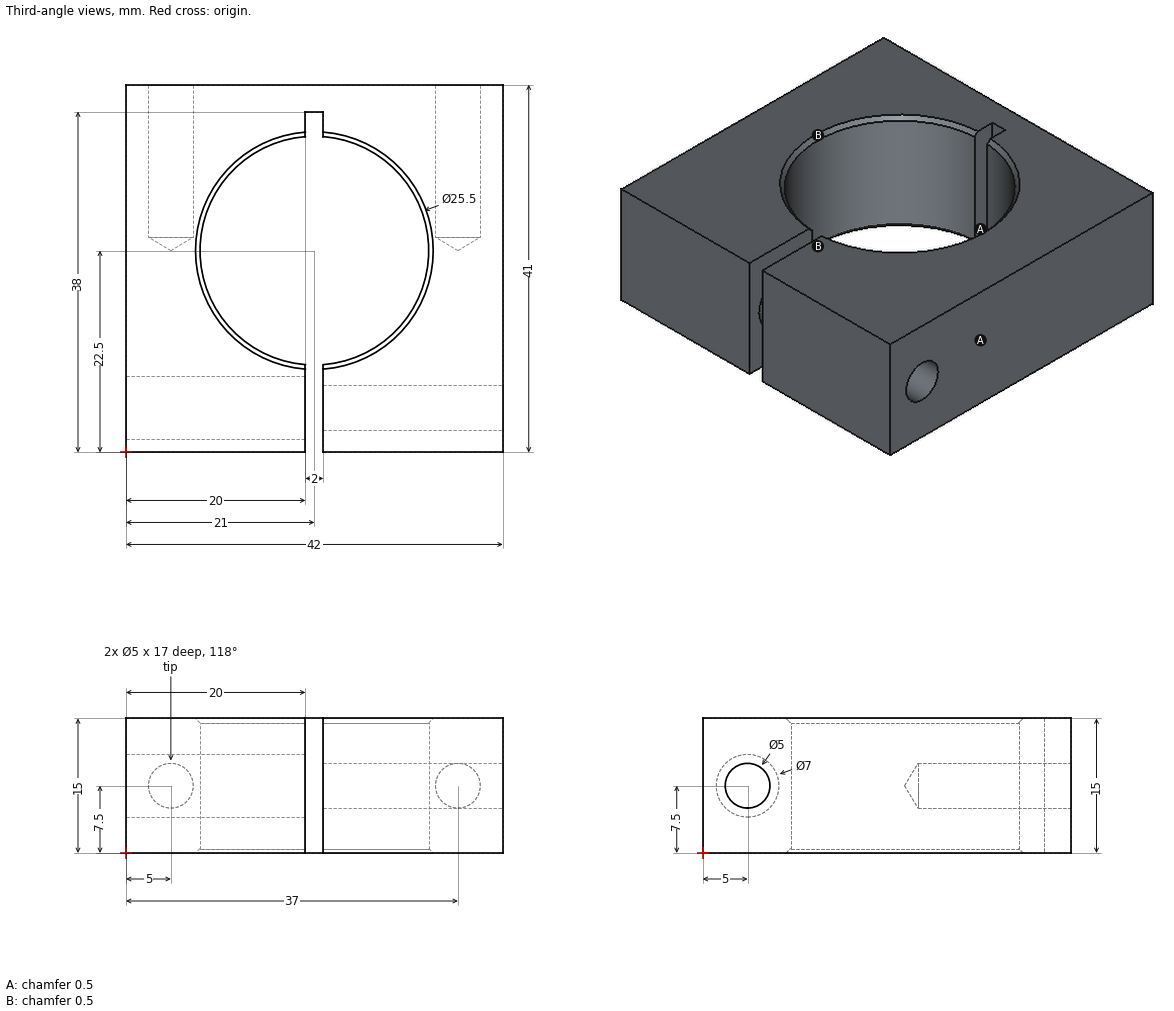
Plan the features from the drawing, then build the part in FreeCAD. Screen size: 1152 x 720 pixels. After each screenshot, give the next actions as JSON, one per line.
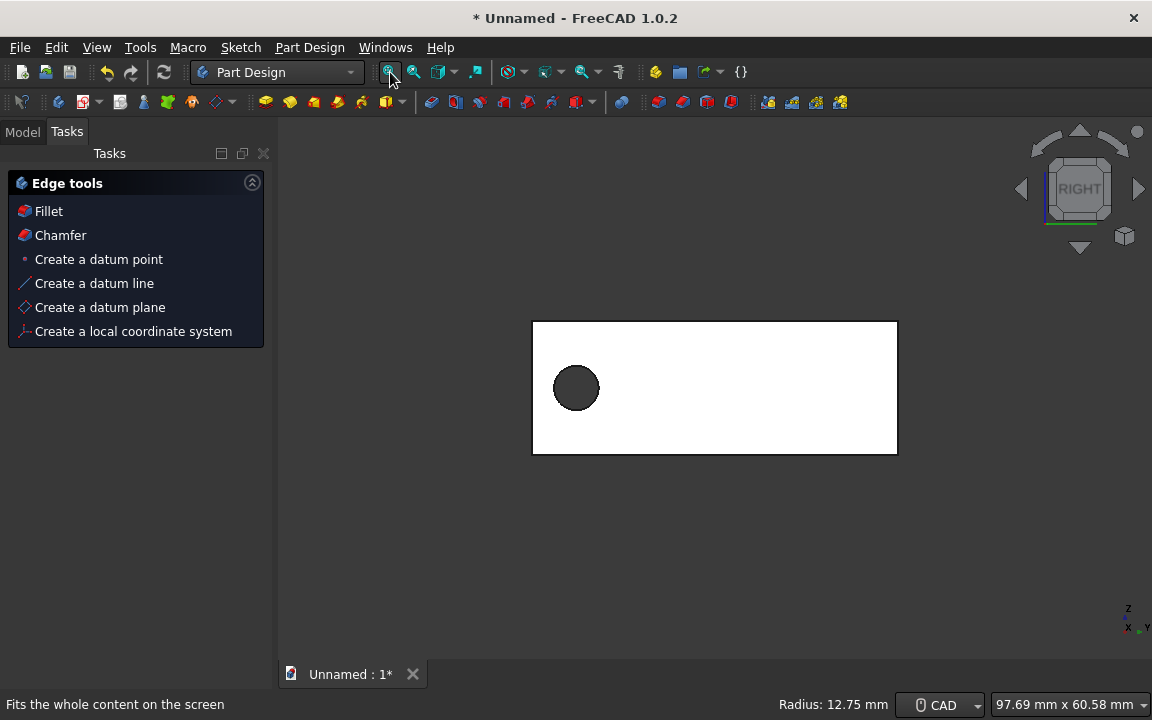
{"action": "left_click", "coordinate": [390, 72]}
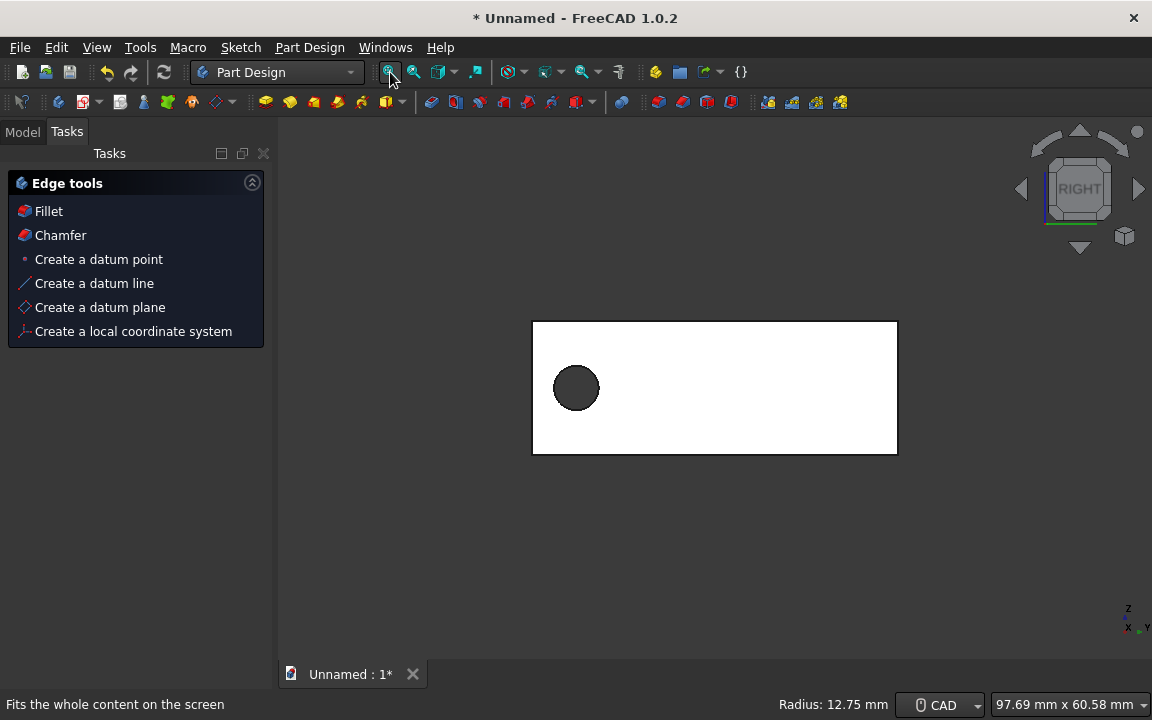
{"action": "key", "text": "5"}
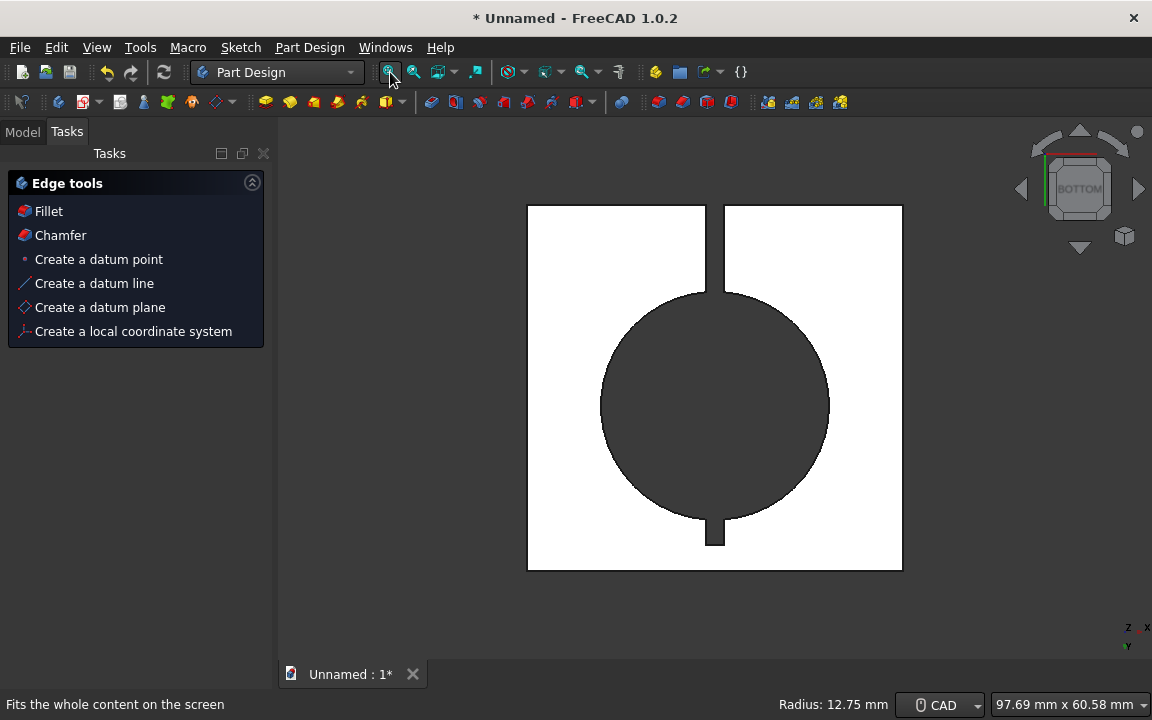
{"action": "left_click", "coordinate": [786, 316], "text": "ctrl"}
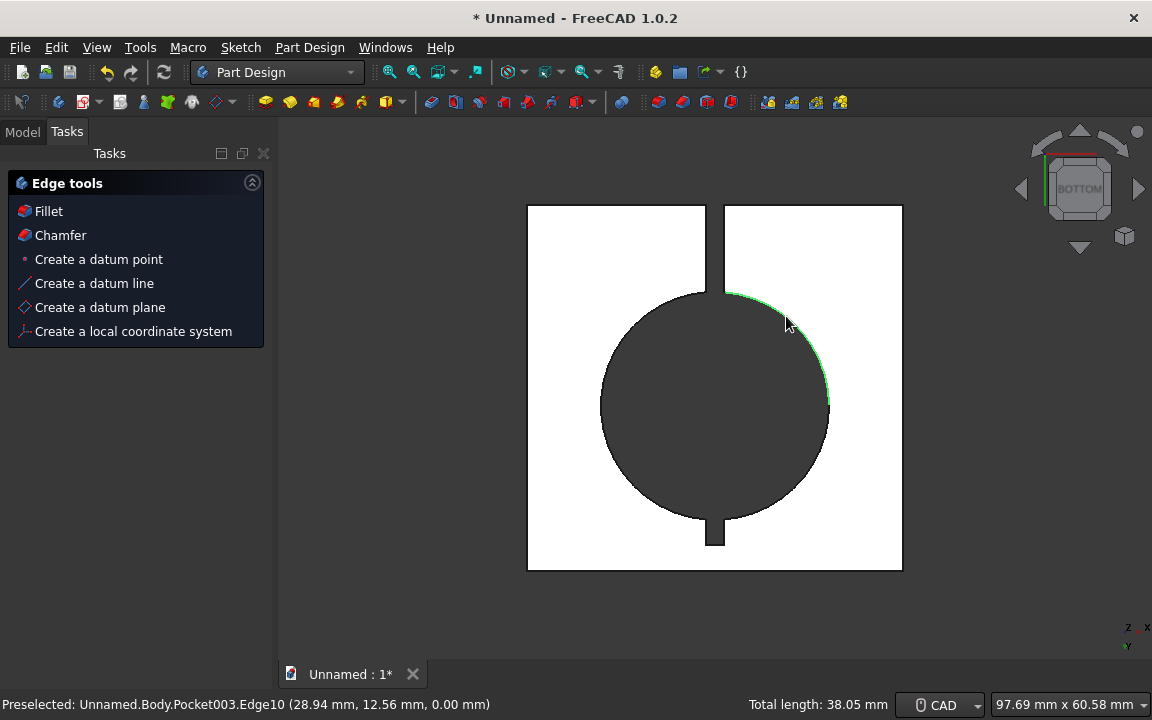
{"action": "left_click", "coordinate": [684, 102]}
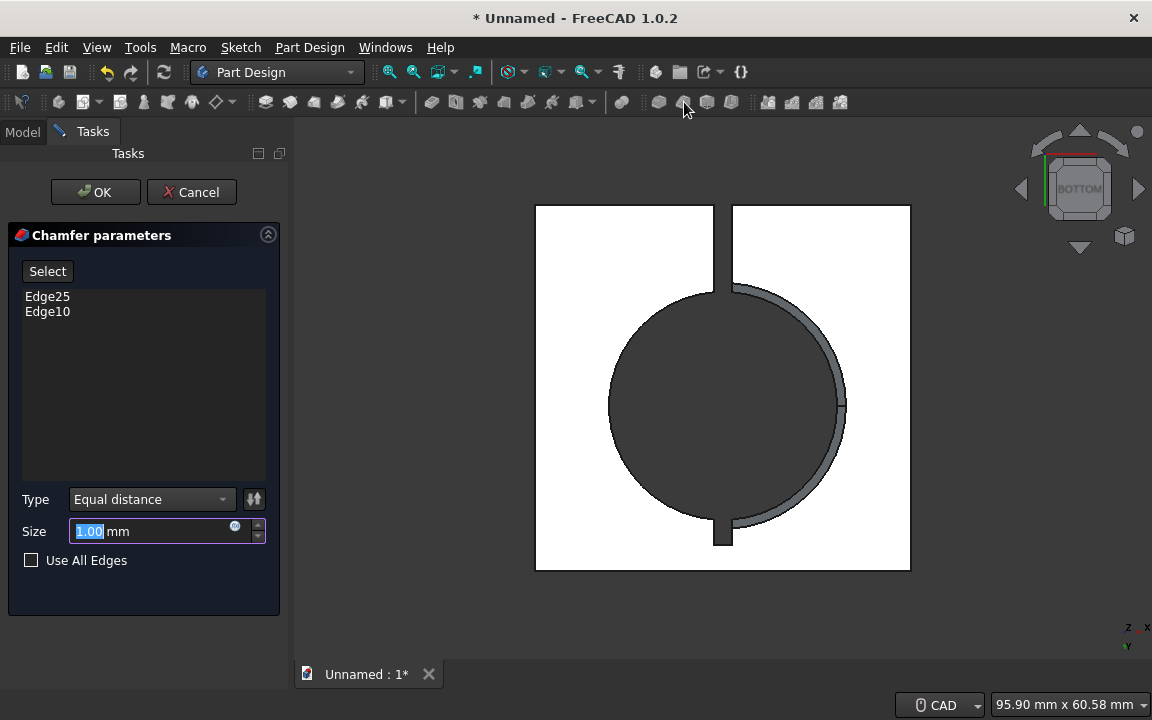
{"action": "type", "text": "0.5"}
{"action": "key", "text": "Tab"}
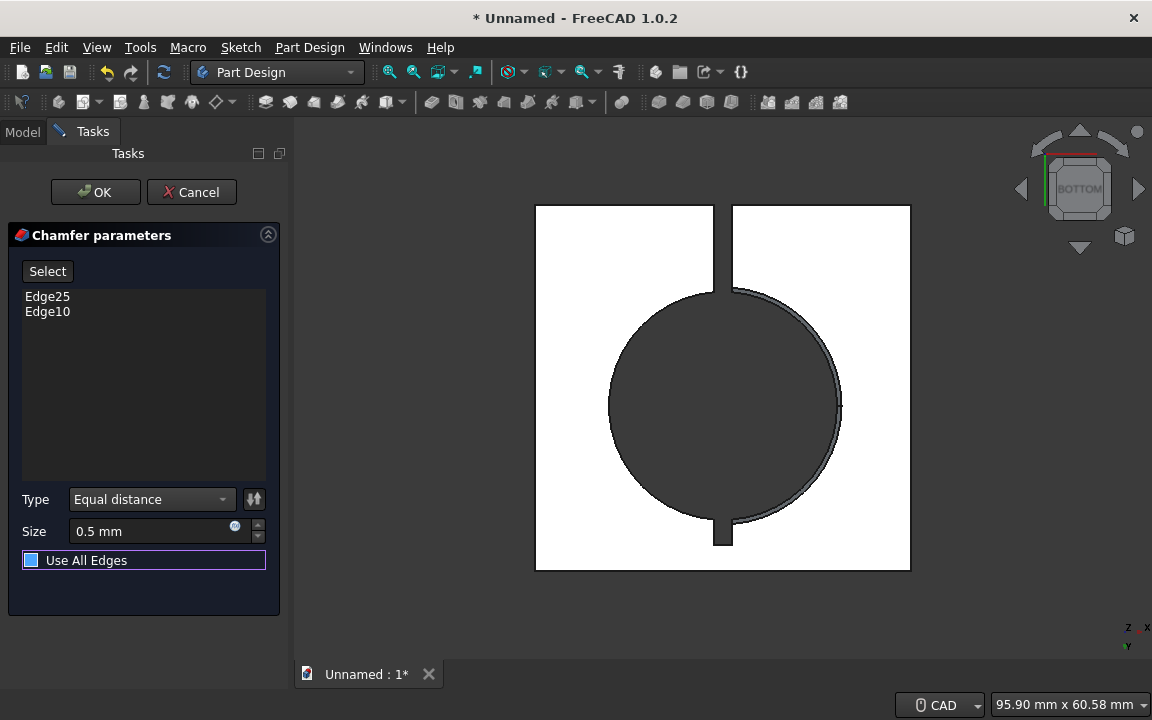
{"action": "left_click", "coordinate": [96, 192]}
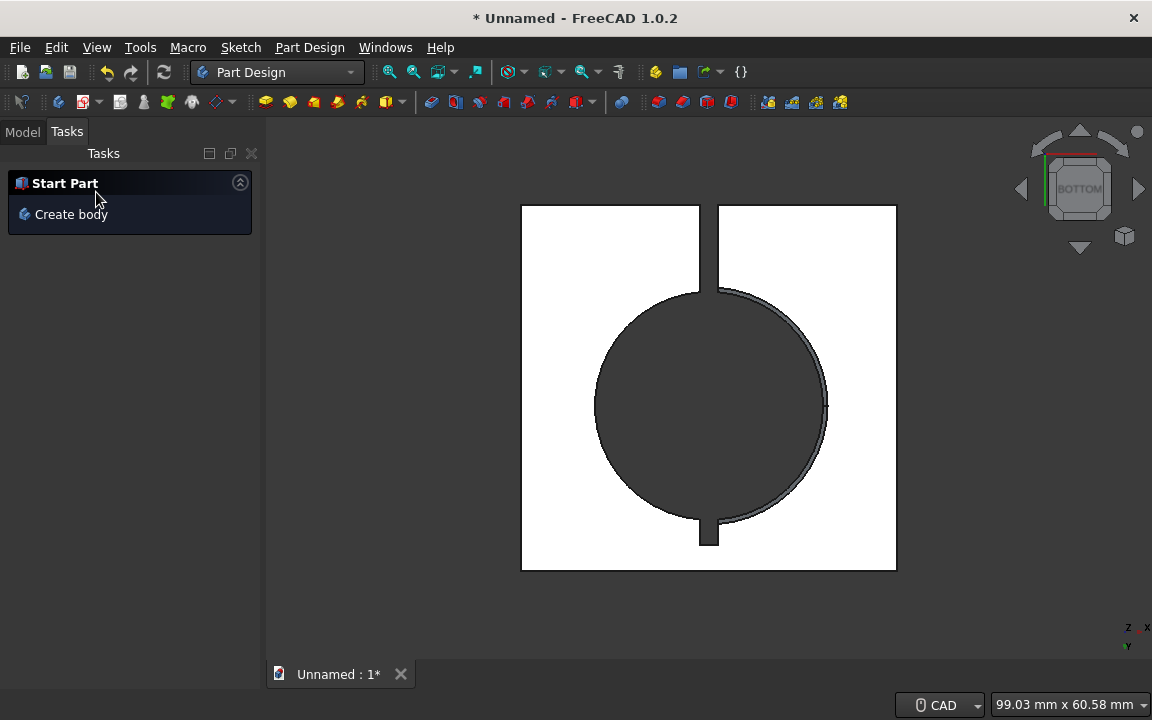
{"action": "left_click", "coordinate": [595, 405]}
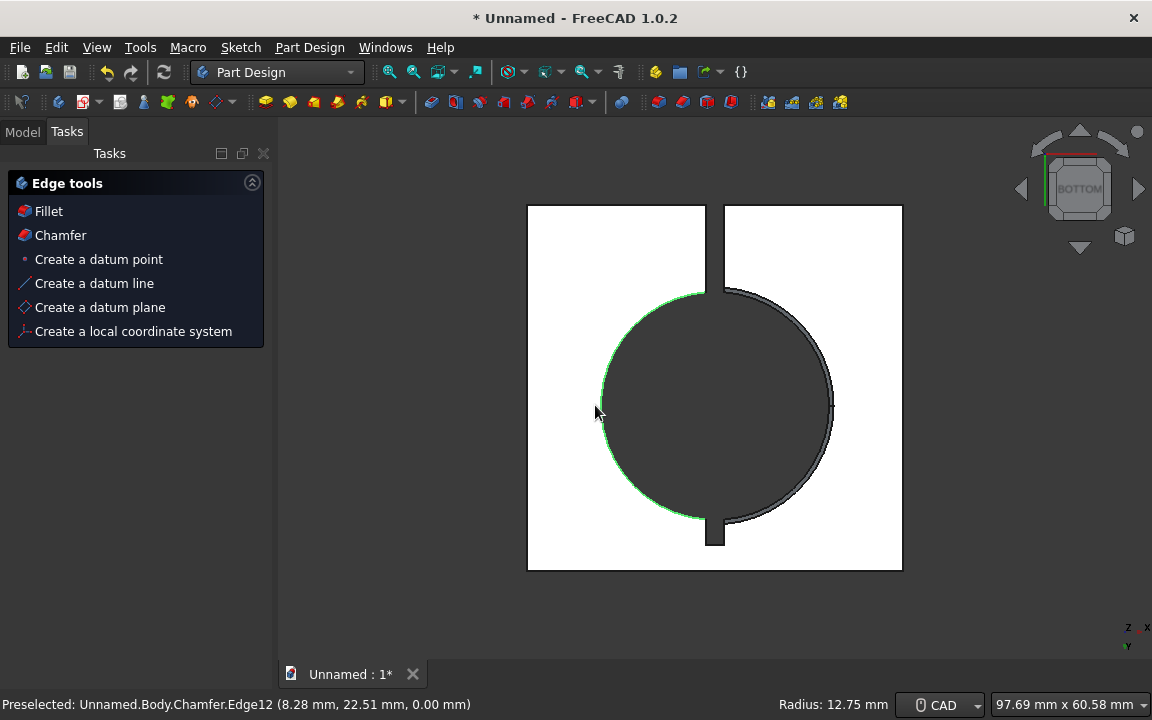
{"action": "key", "text": "0"}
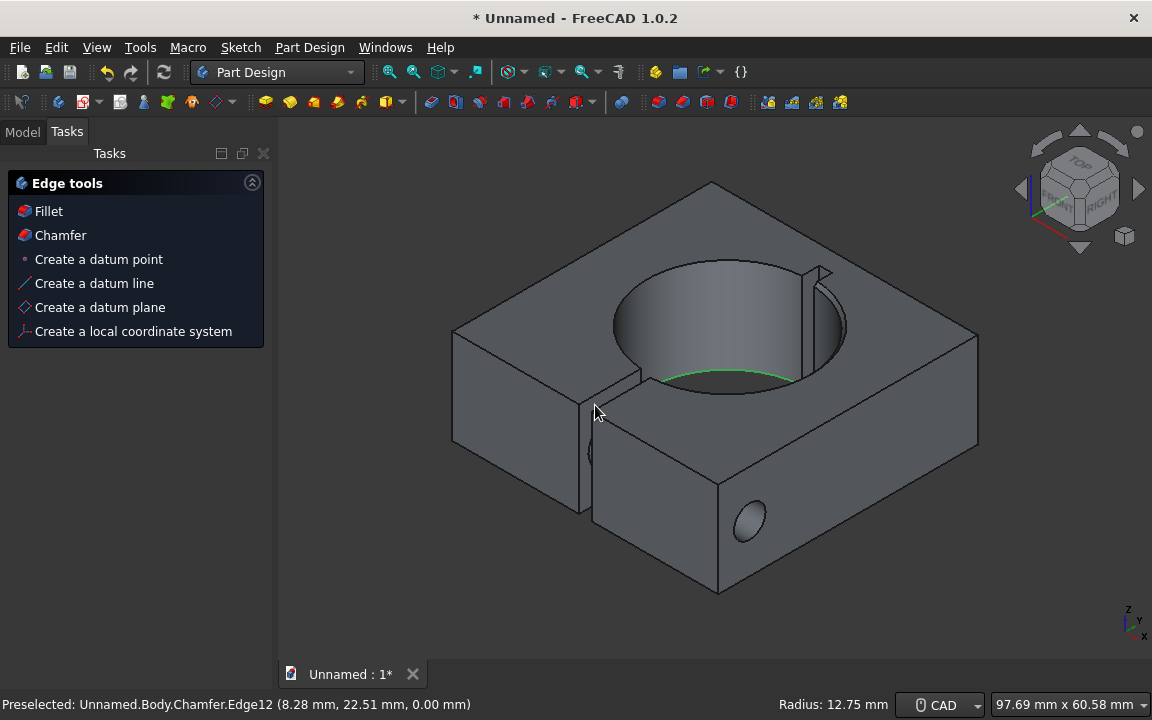
{"action": "left_click", "coordinate": [647, 278], "text": "ctrl"}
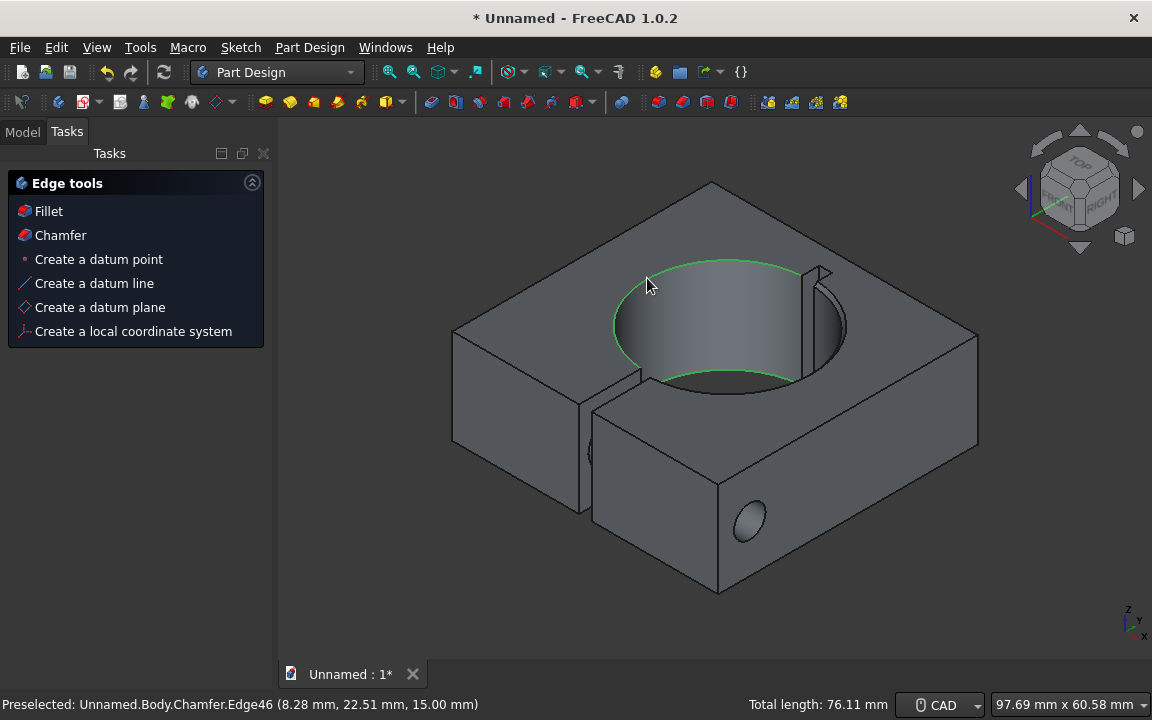
{"action": "left_click", "coordinate": [684, 102]}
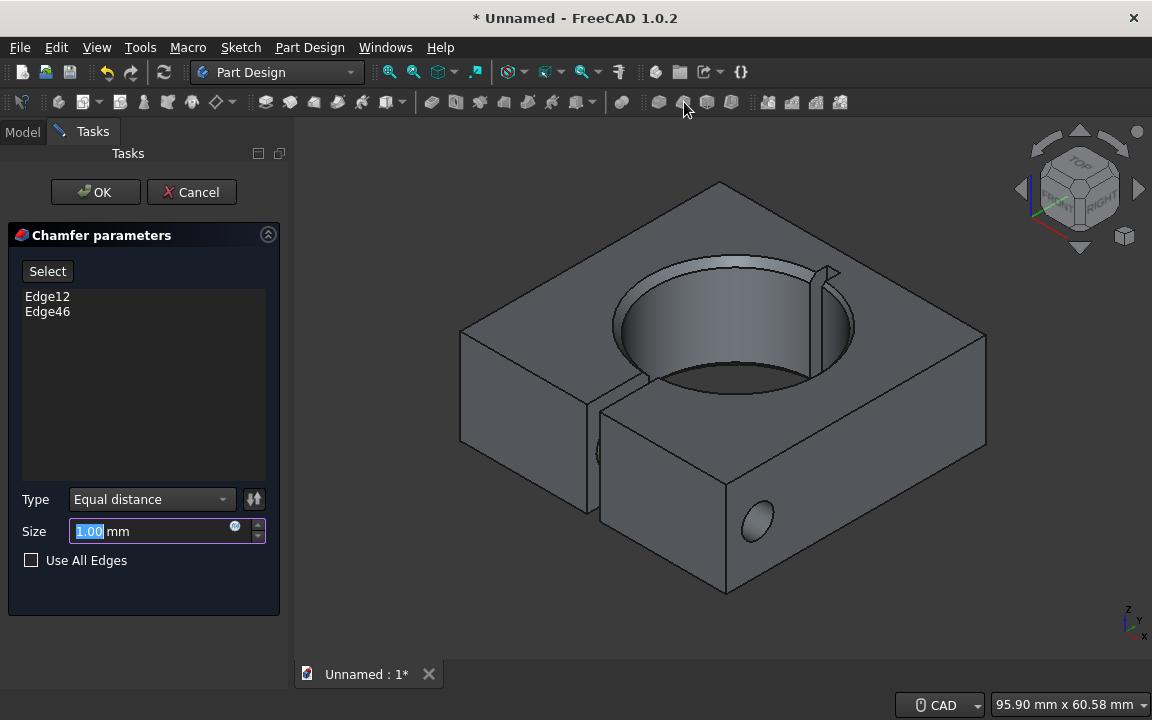
{"action": "type", "text": "0.5"}
{"action": "key", "text": "Tab"}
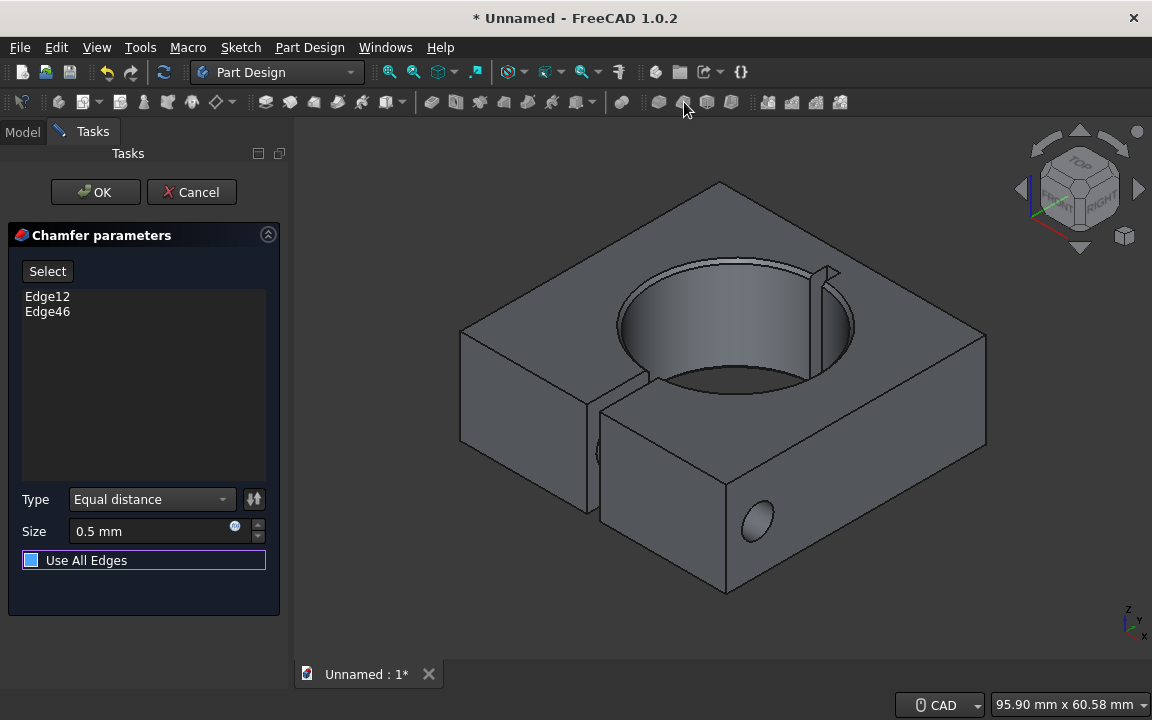
{"action": "left_click", "coordinate": [96, 192]}